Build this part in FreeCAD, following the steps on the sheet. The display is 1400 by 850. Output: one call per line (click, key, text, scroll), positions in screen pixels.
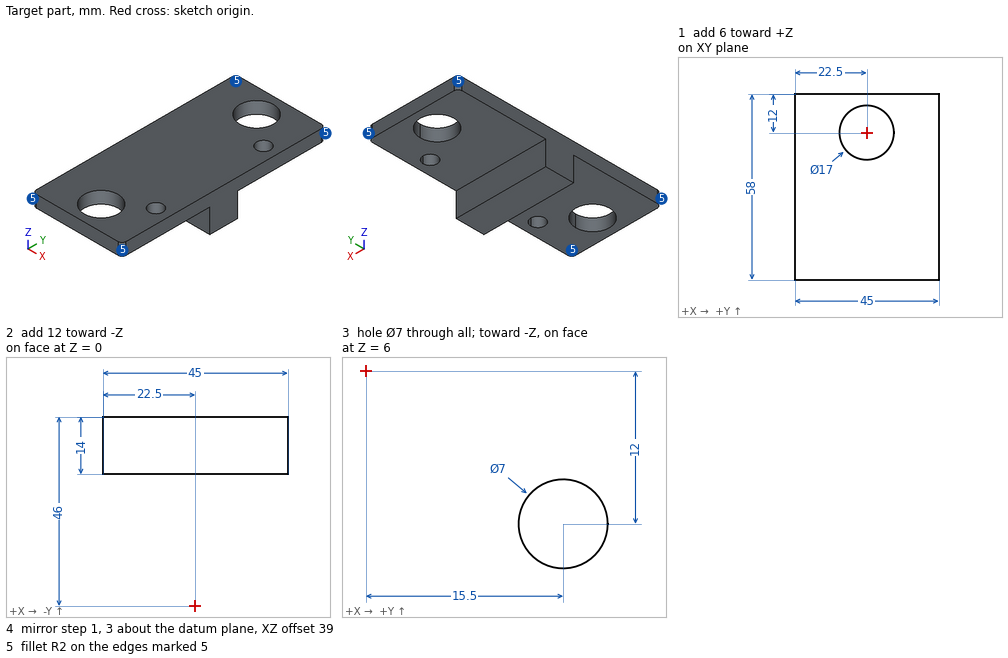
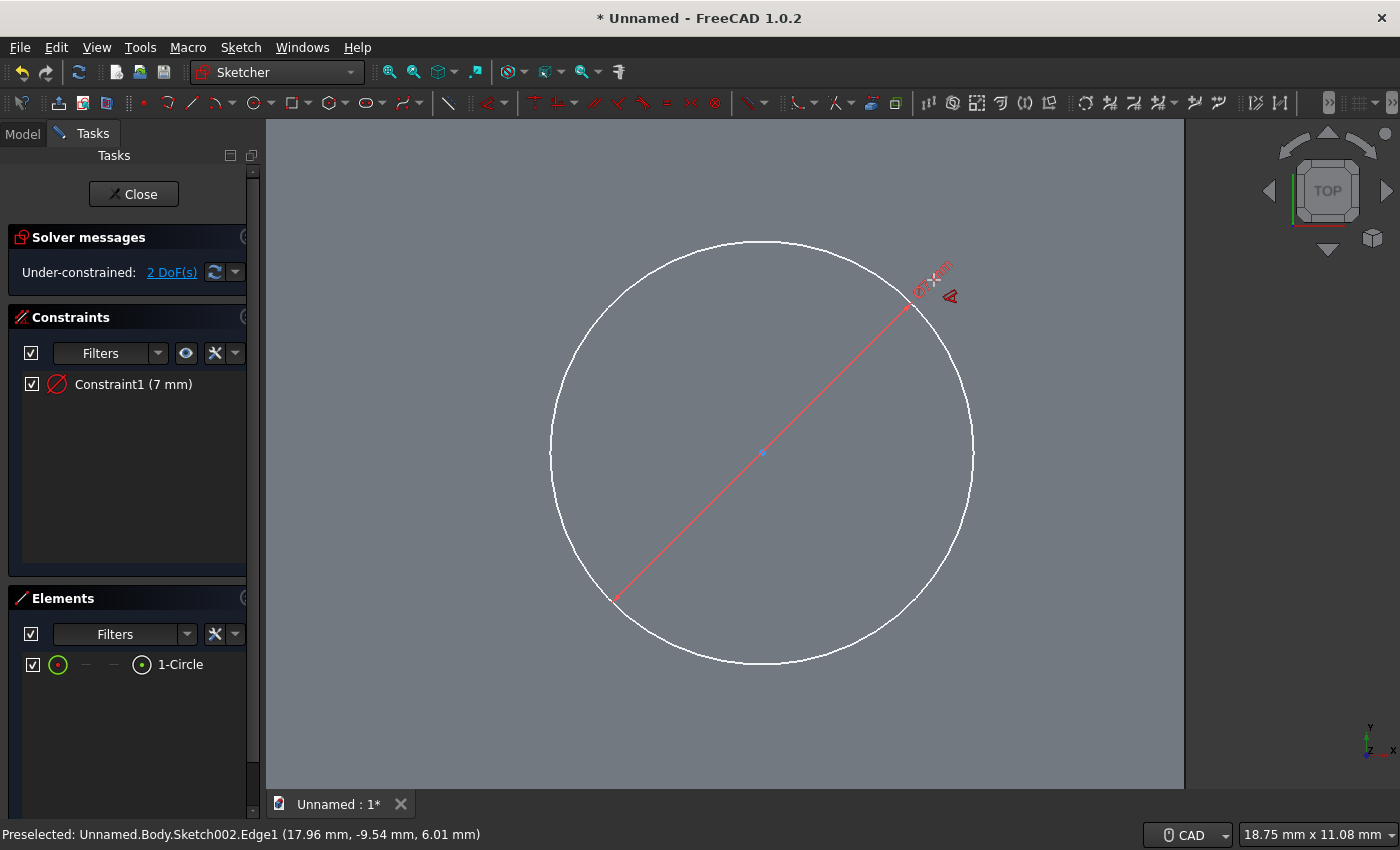
click(762, 453)
click(796, 300)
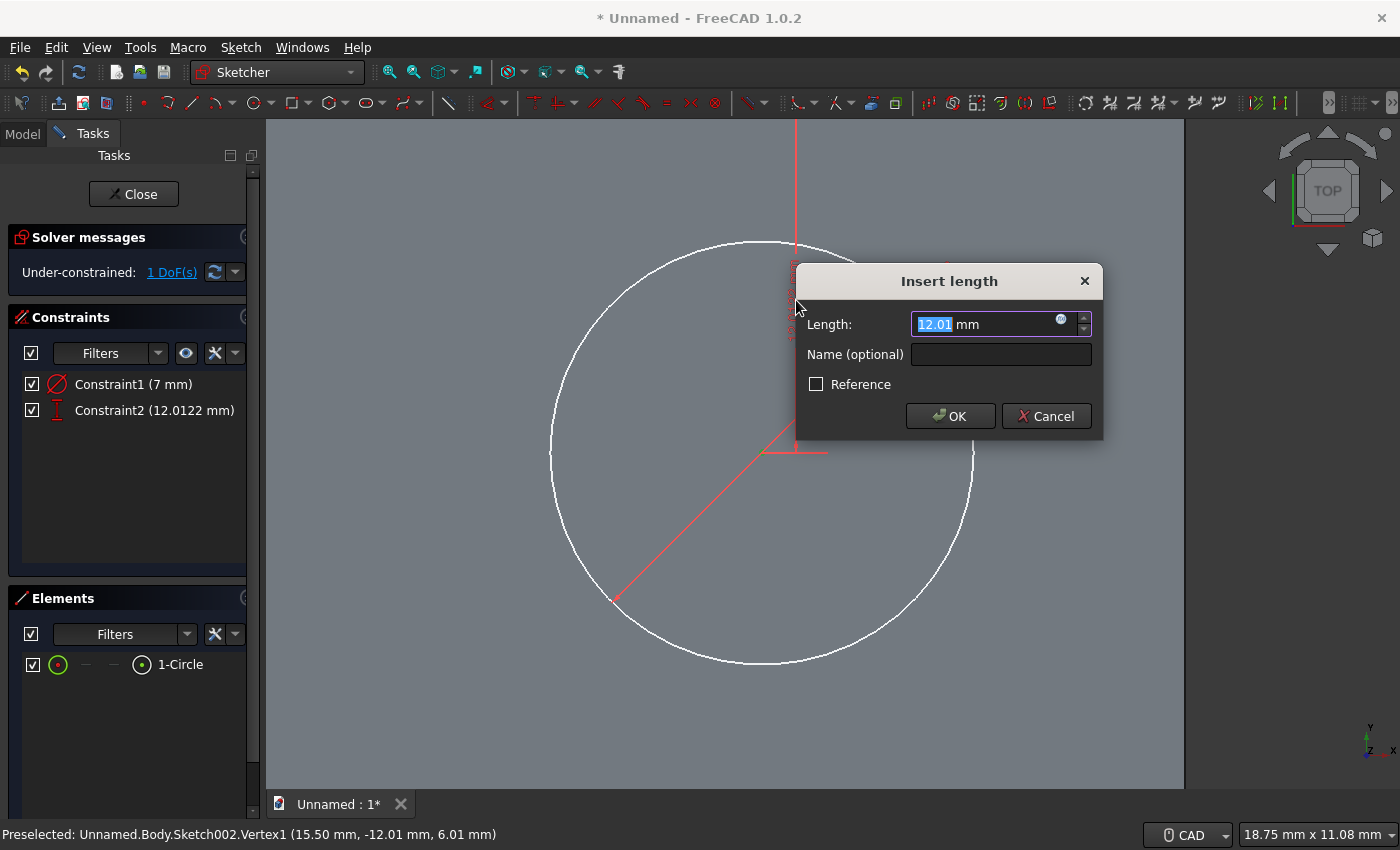
text(12)
key(Return)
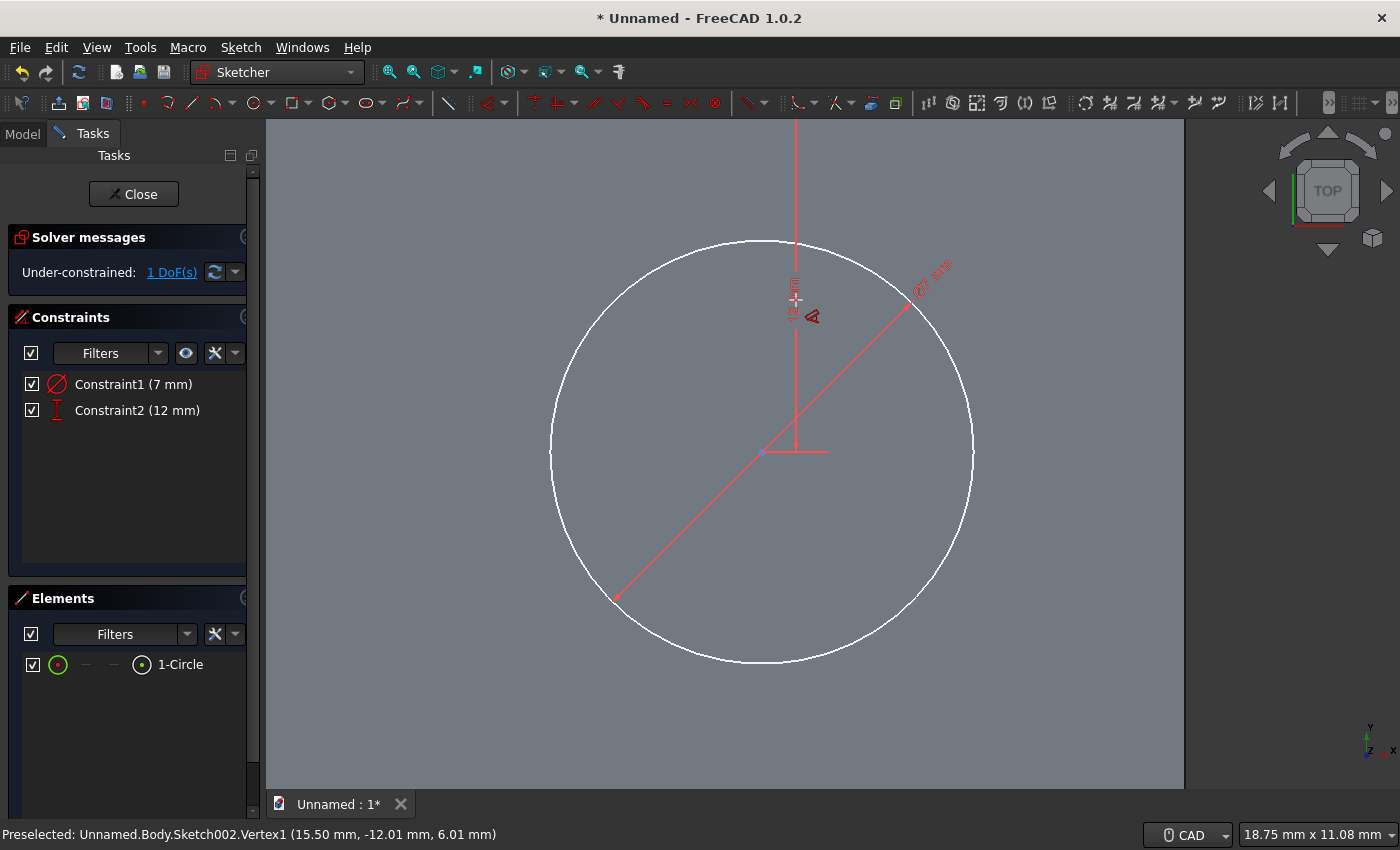
click(762, 452)
click(528, 486)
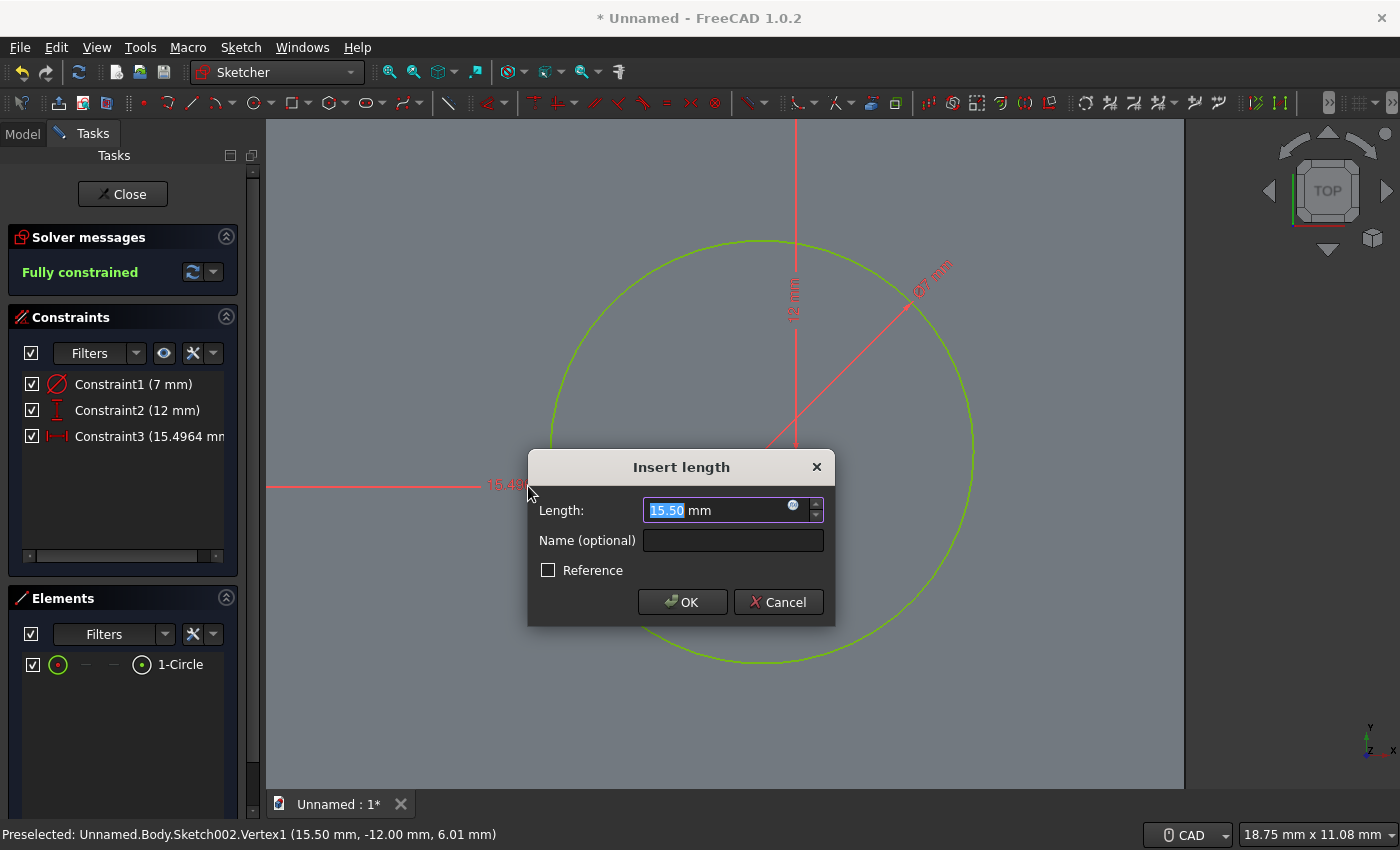
text(15.5)
key(Return)
key(Escape)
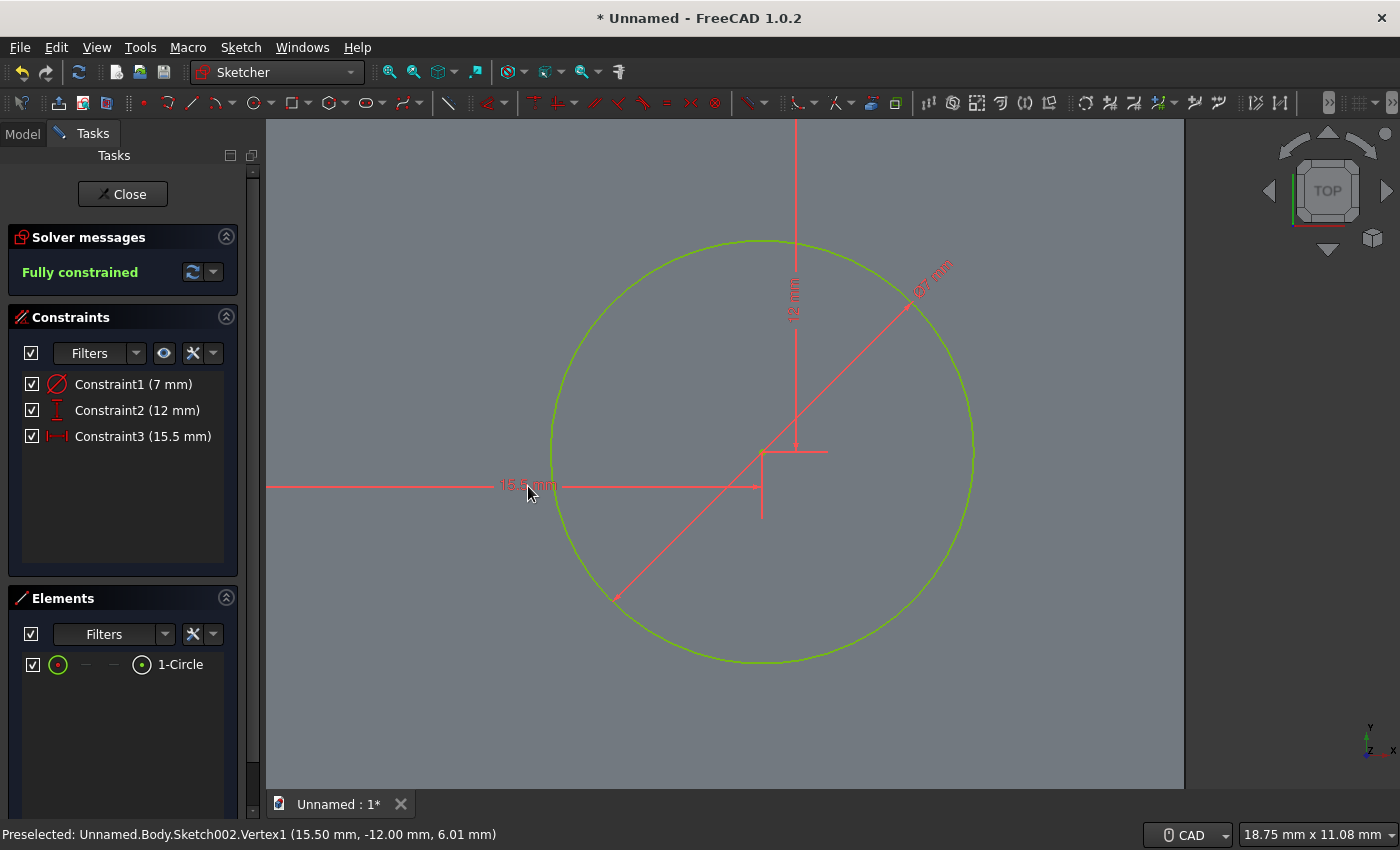
click(123, 194)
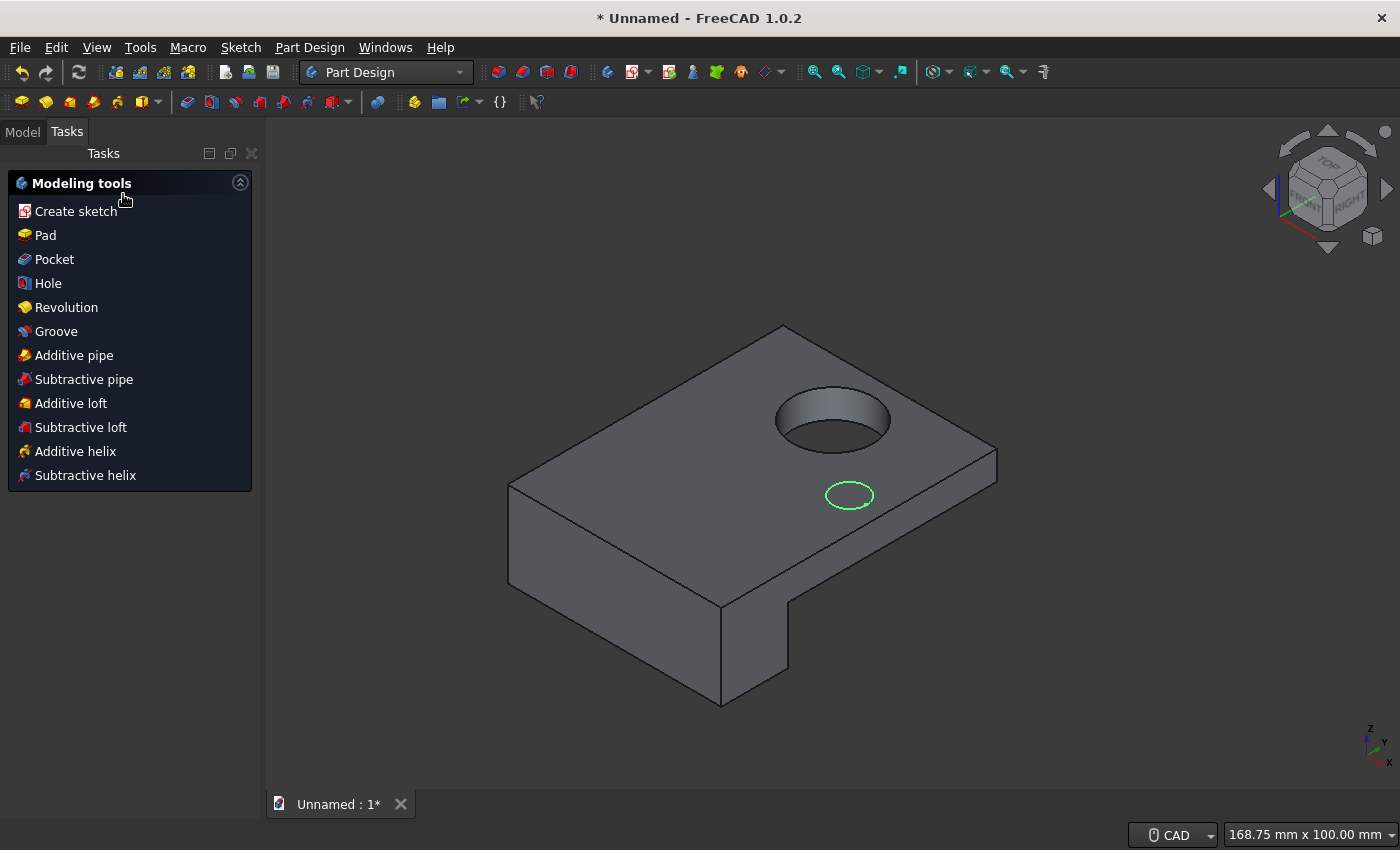
click(212, 102)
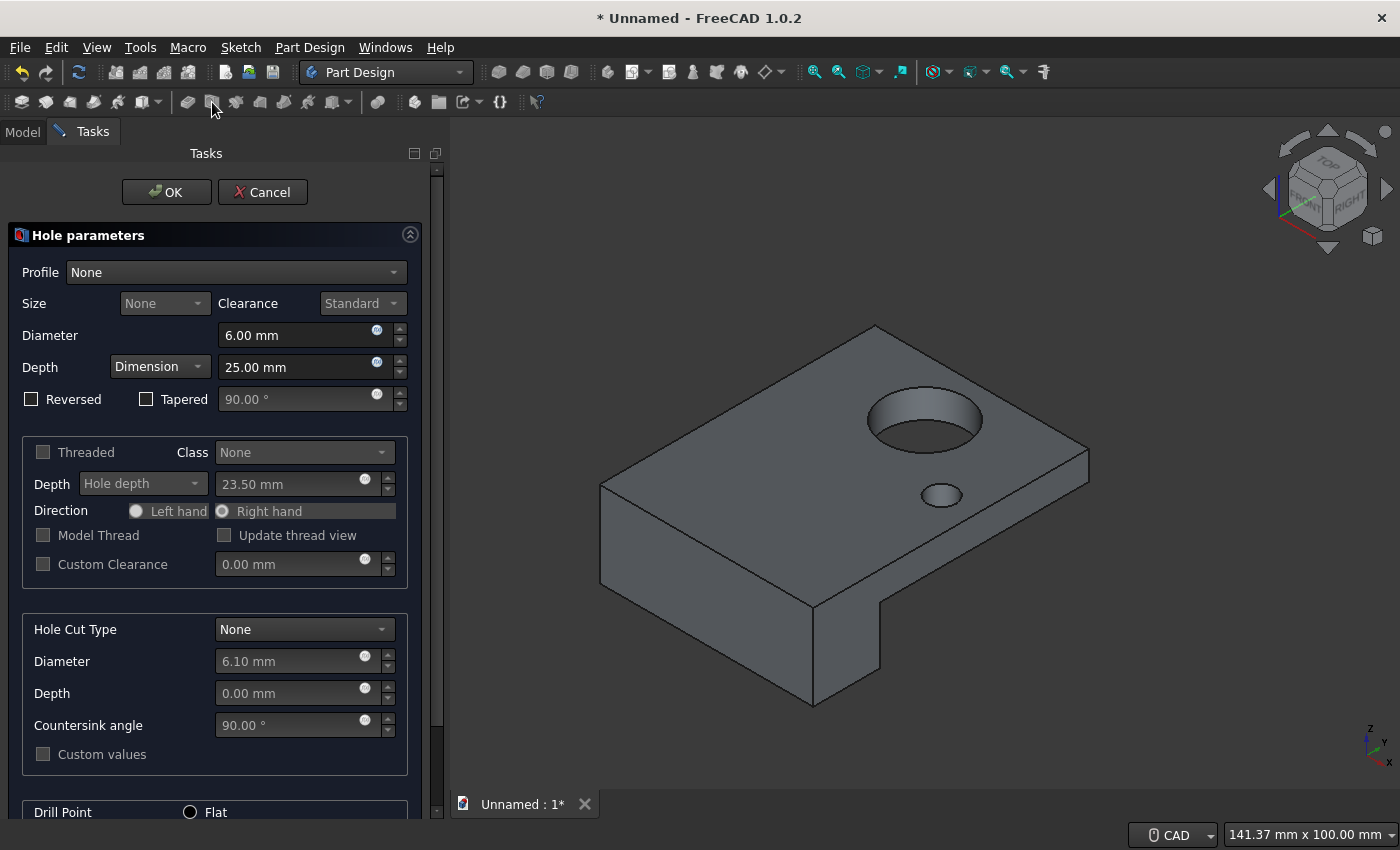
triple_click(305, 335)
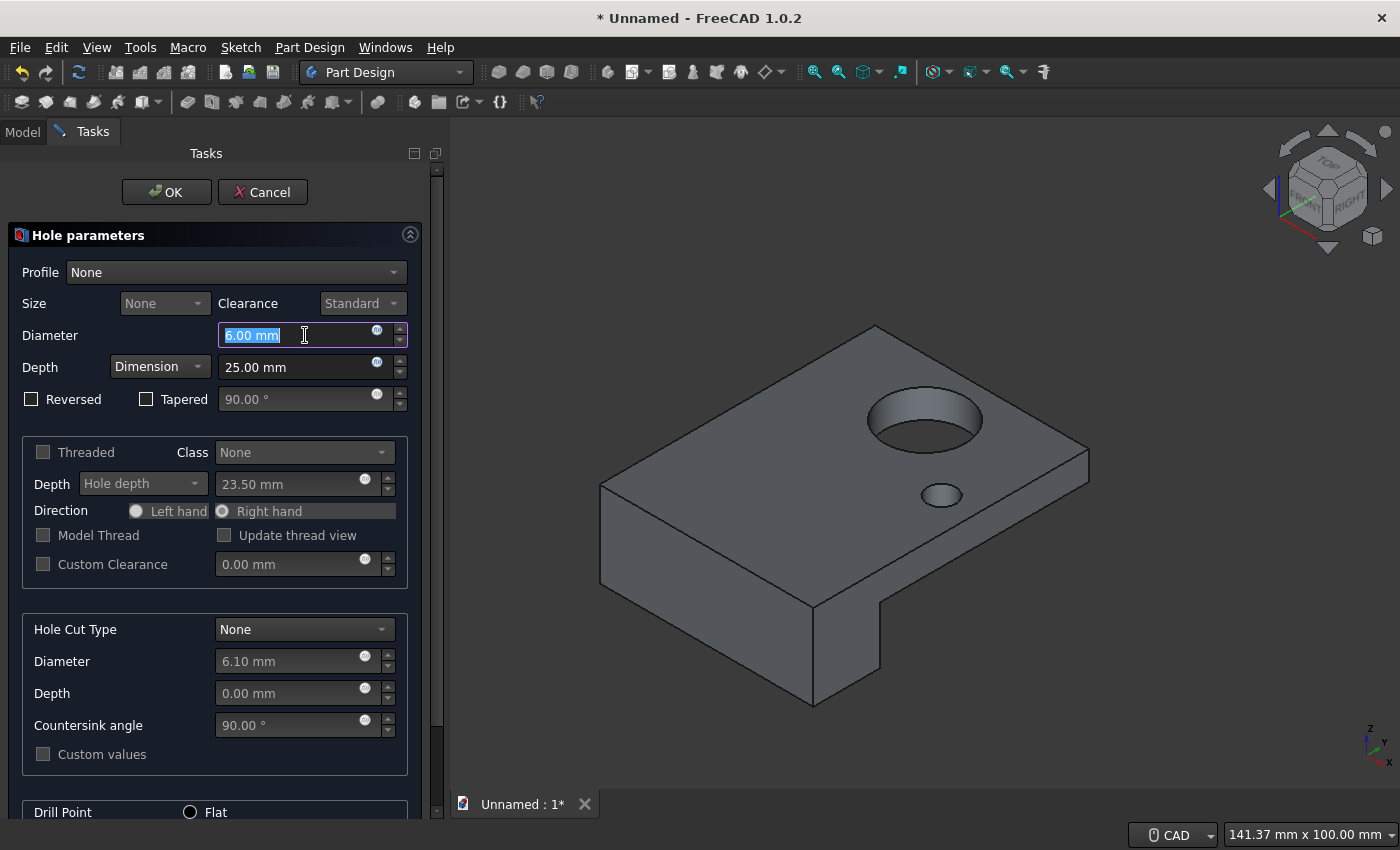
text(7)
key(Tab)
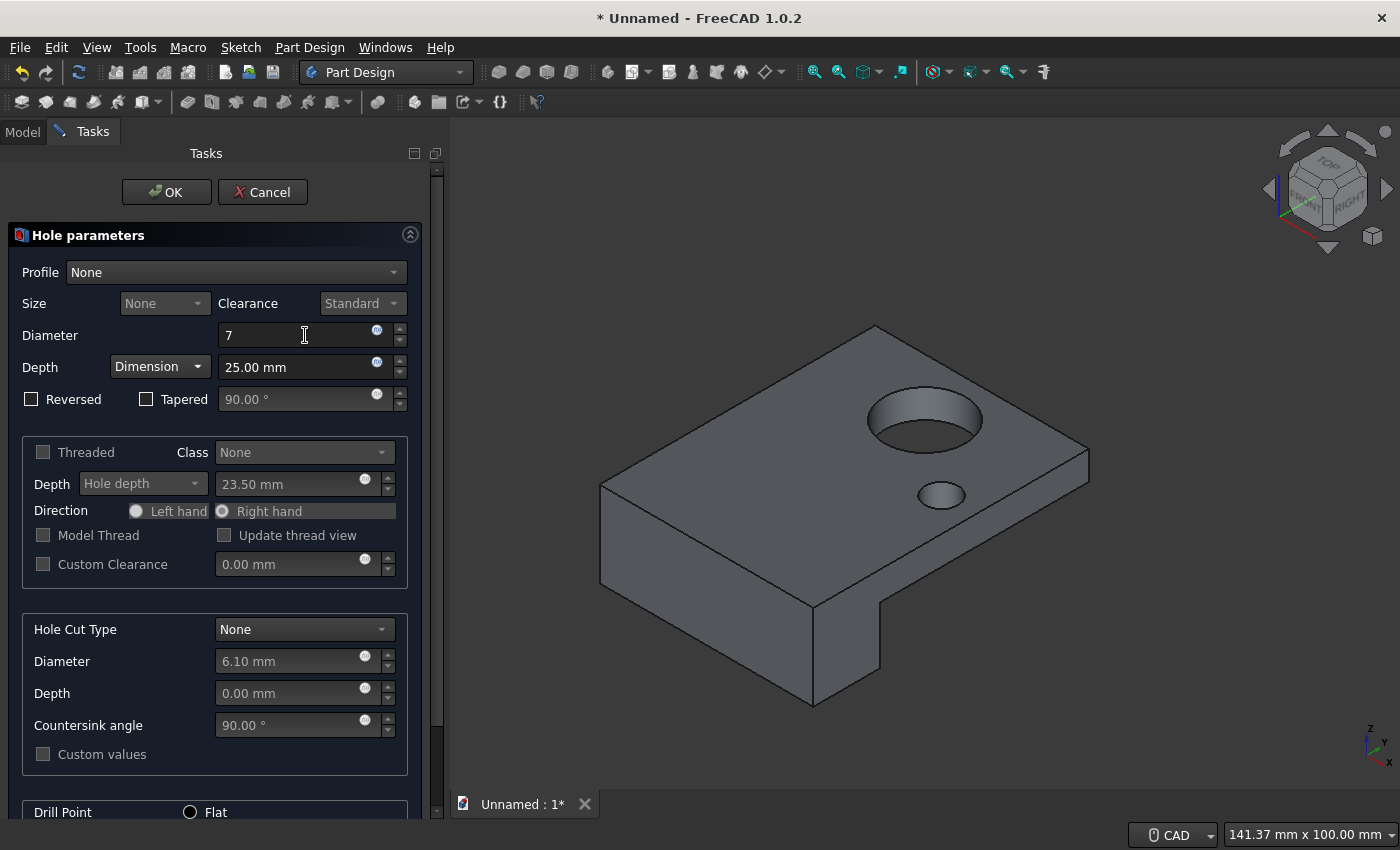
click(161, 366)